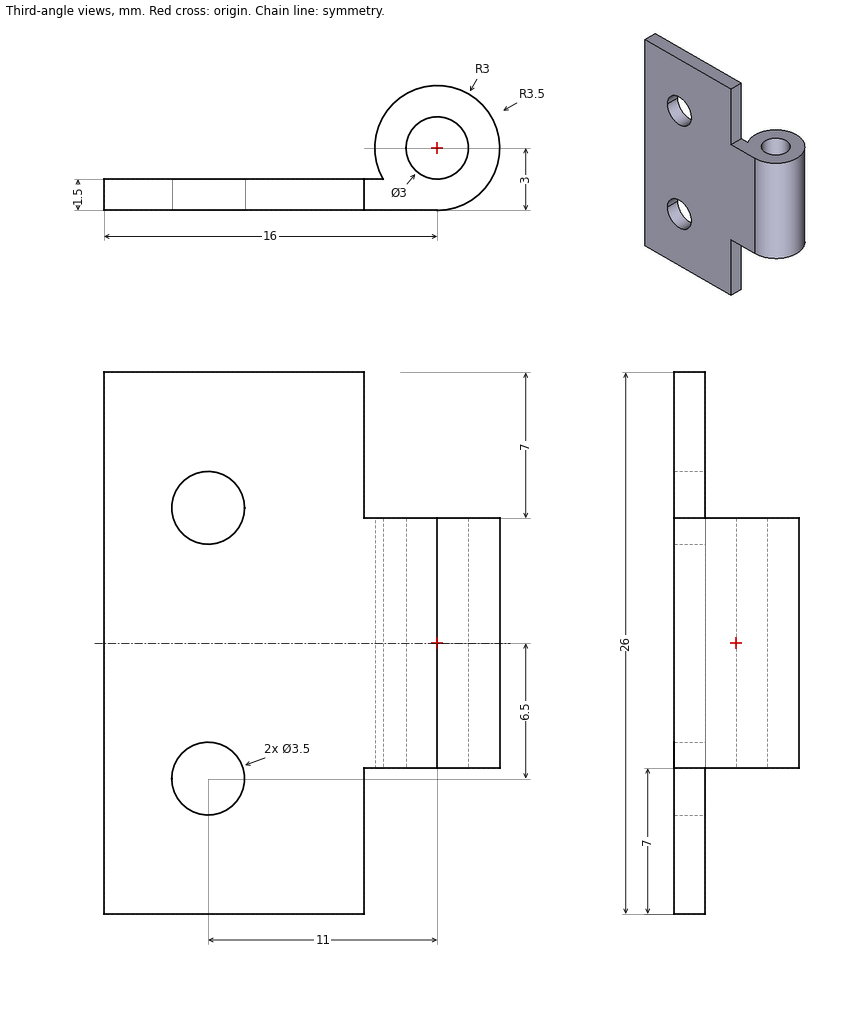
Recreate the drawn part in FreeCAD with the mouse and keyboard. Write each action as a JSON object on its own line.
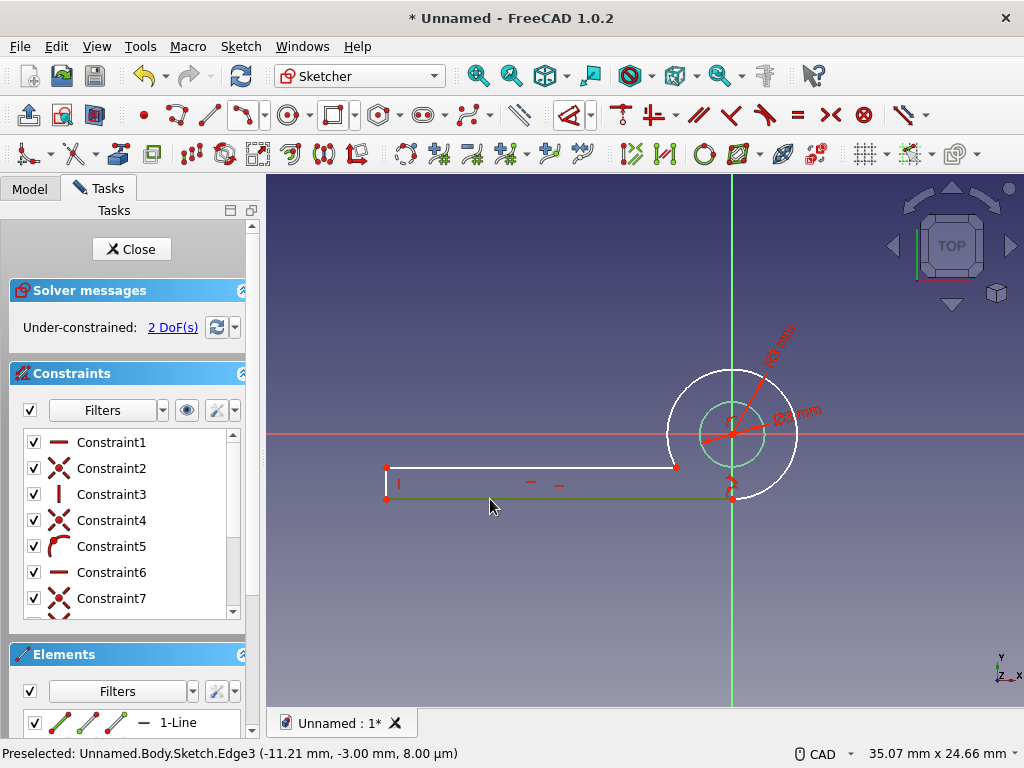
{"action": "left_click", "coordinate": [590, 116]}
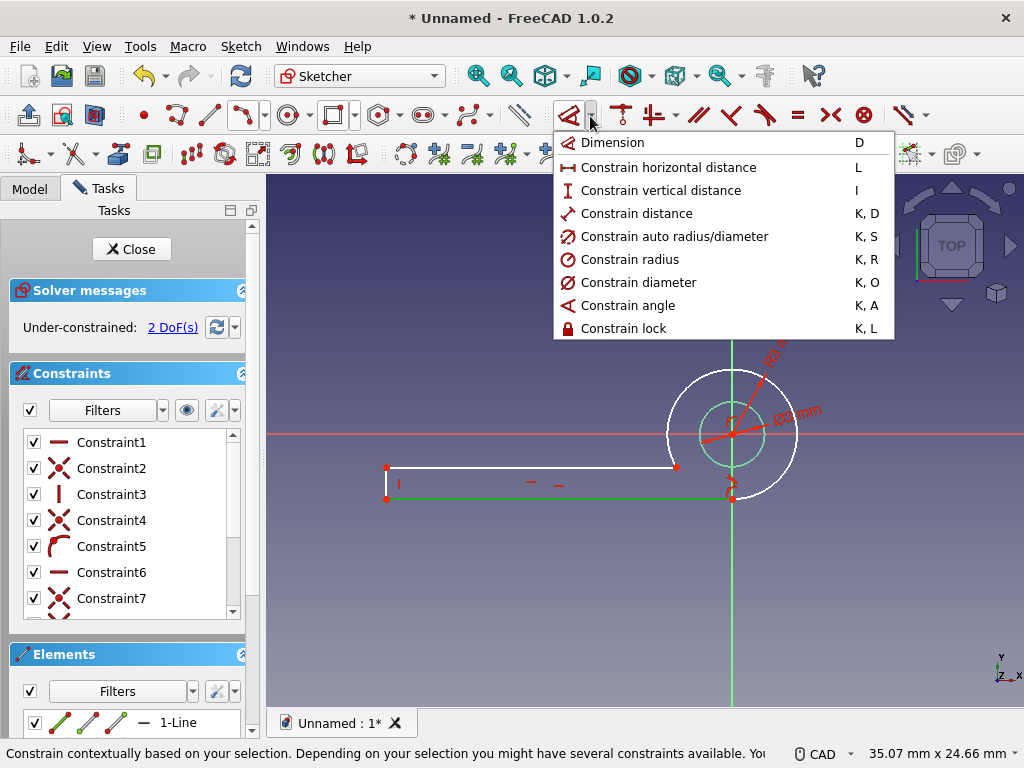
{"action": "left_click", "coordinate": [724, 168]}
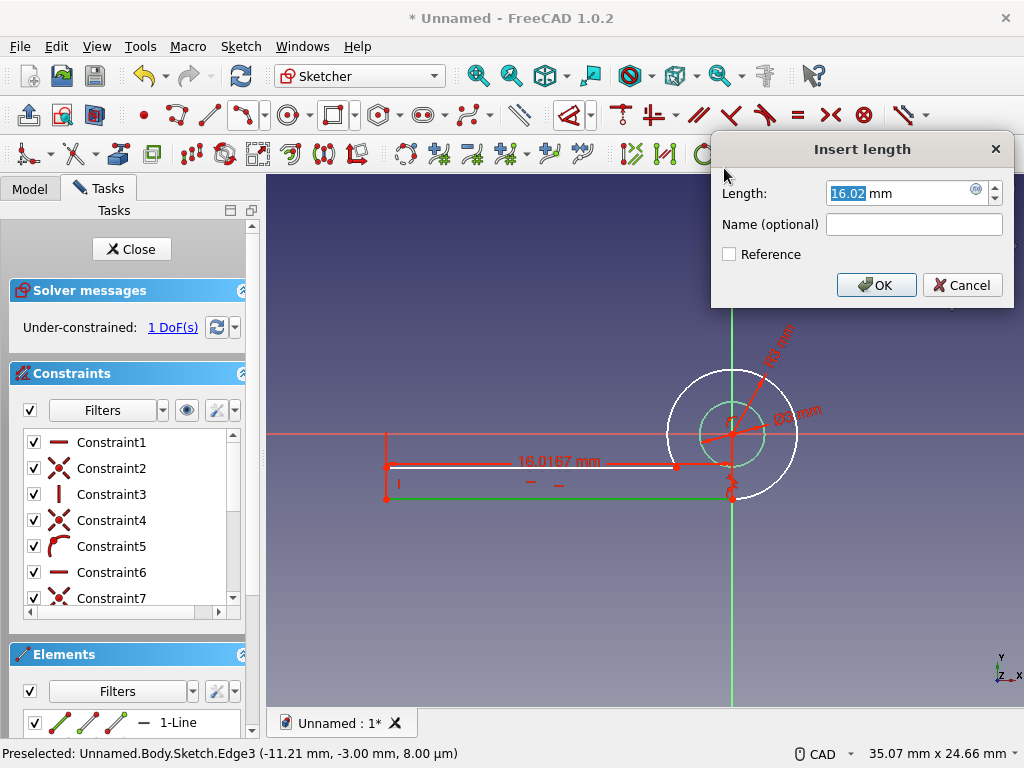
{"action": "type", "text": "16"}
{"action": "key", "text": "Return"}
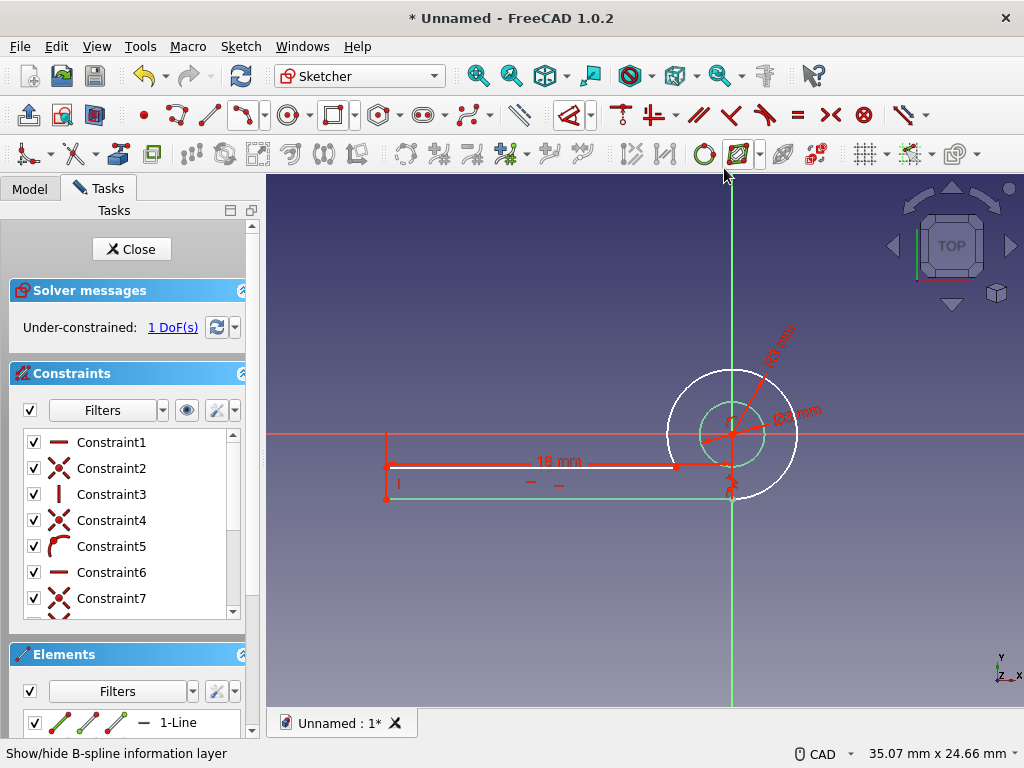
{"action": "scroll", "coordinate": [386, 477], "scroll_direction": "up", "scroll_amount": 2}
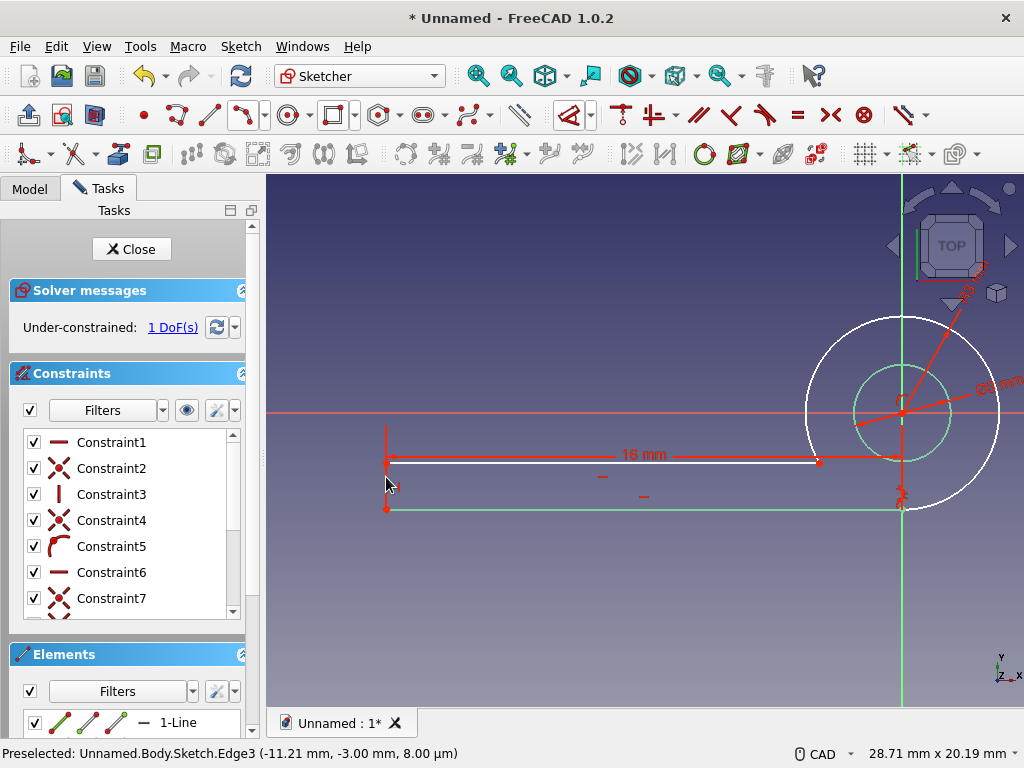
{"action": "left_click", "coordinate": [386, 477]}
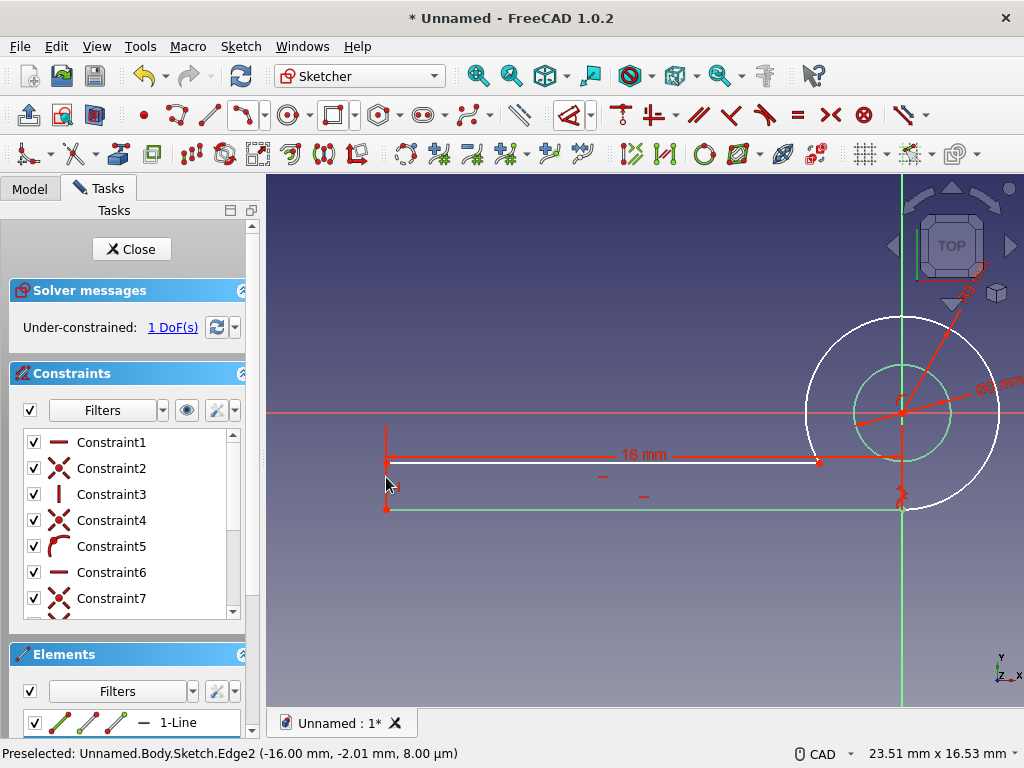
{"action": "left_click", "coordinate": [590, 116]}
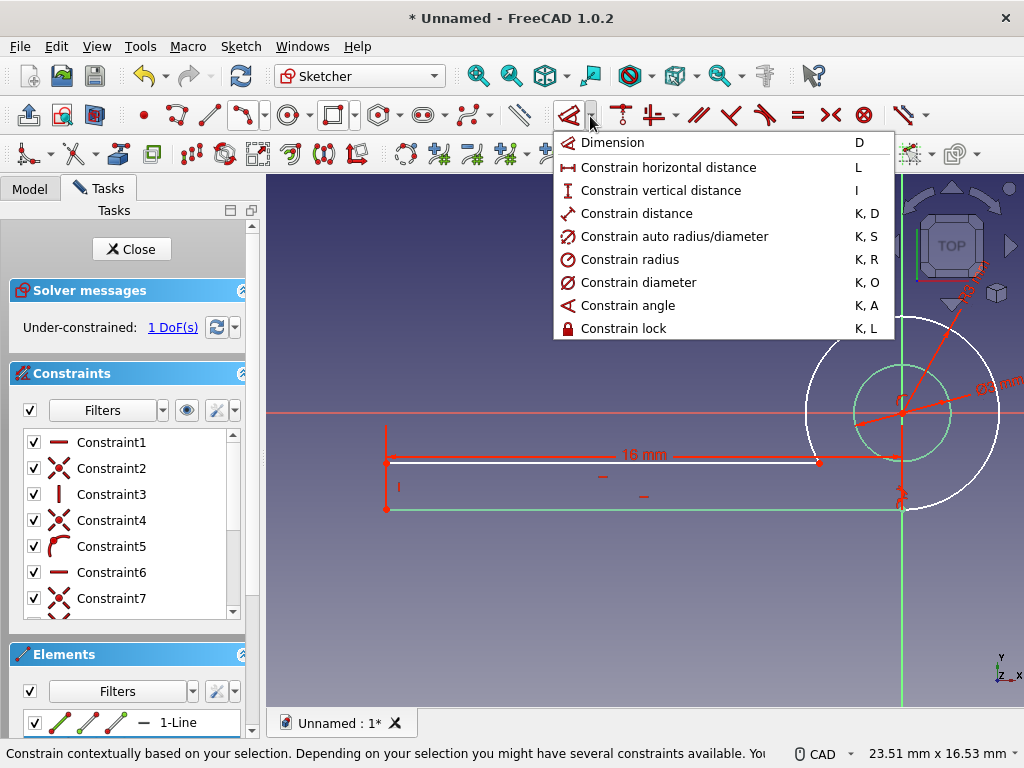
{"action": "left_click", "coordinate": [724, 190]}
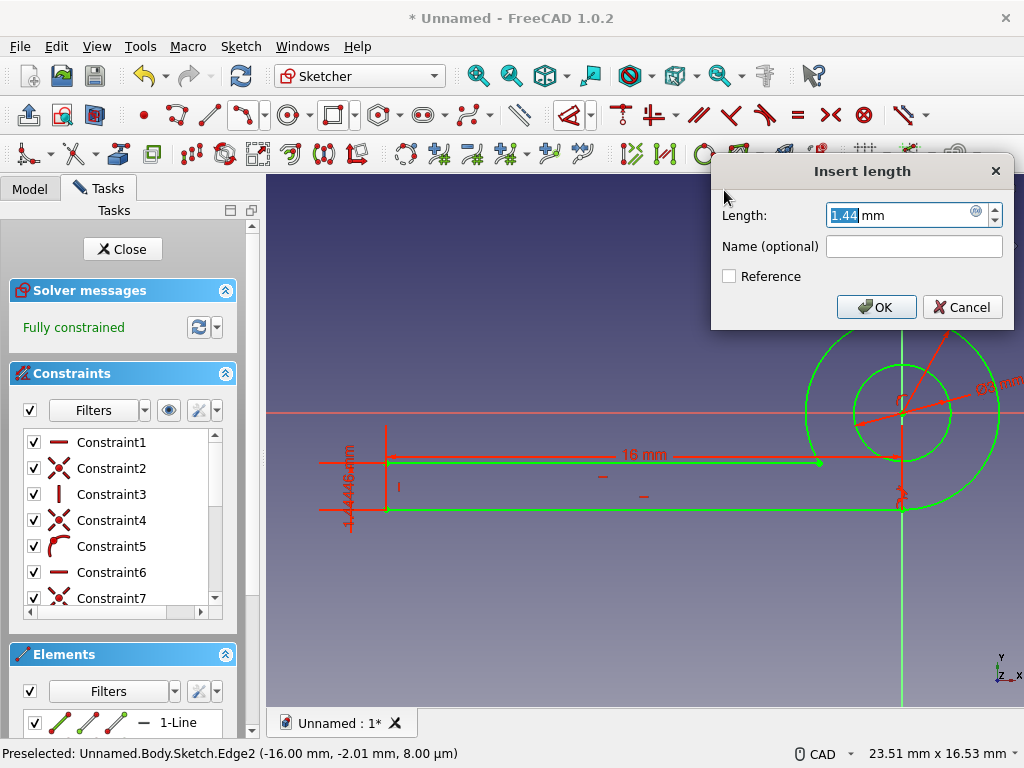
{"action": "type", "text": "1.5"}
{"action": "key", "text": "Return"}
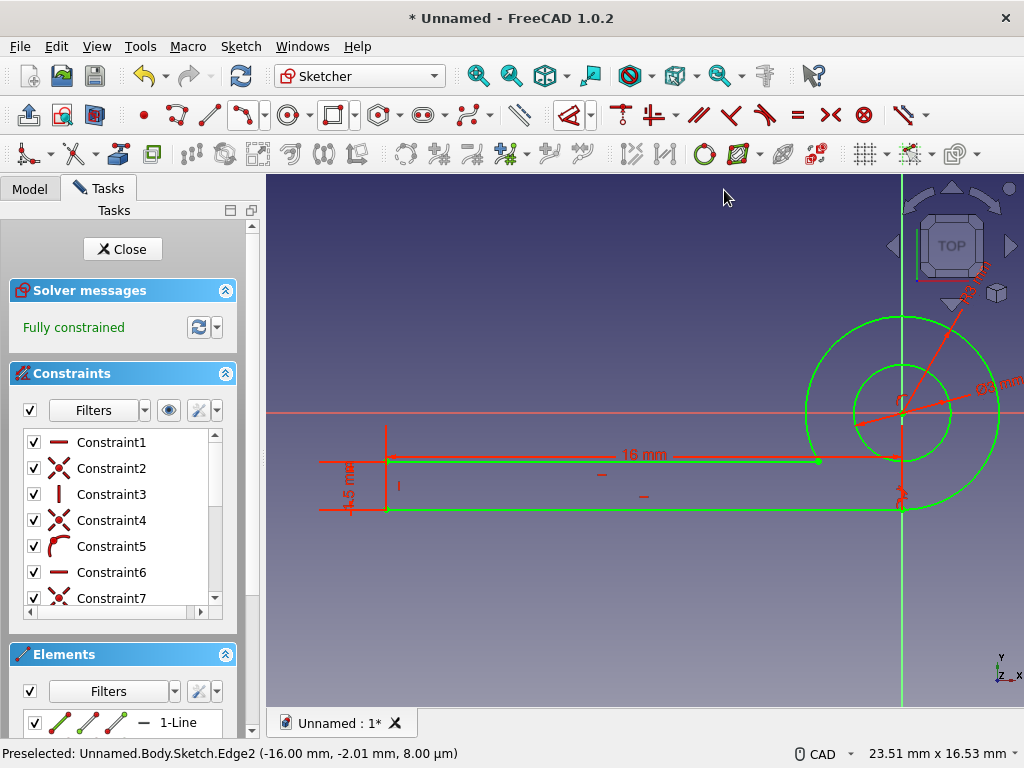
{"action": "left_click", "coordinate": [123, 249]}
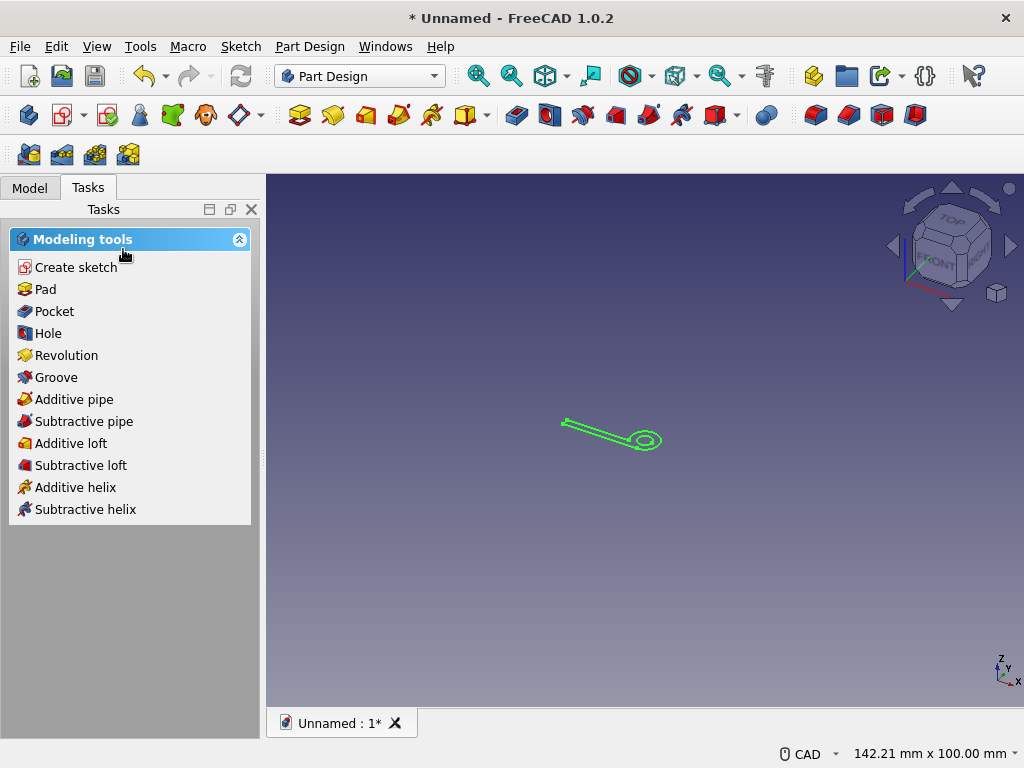
{"action": "left_click", "coordinate": [300, 116]}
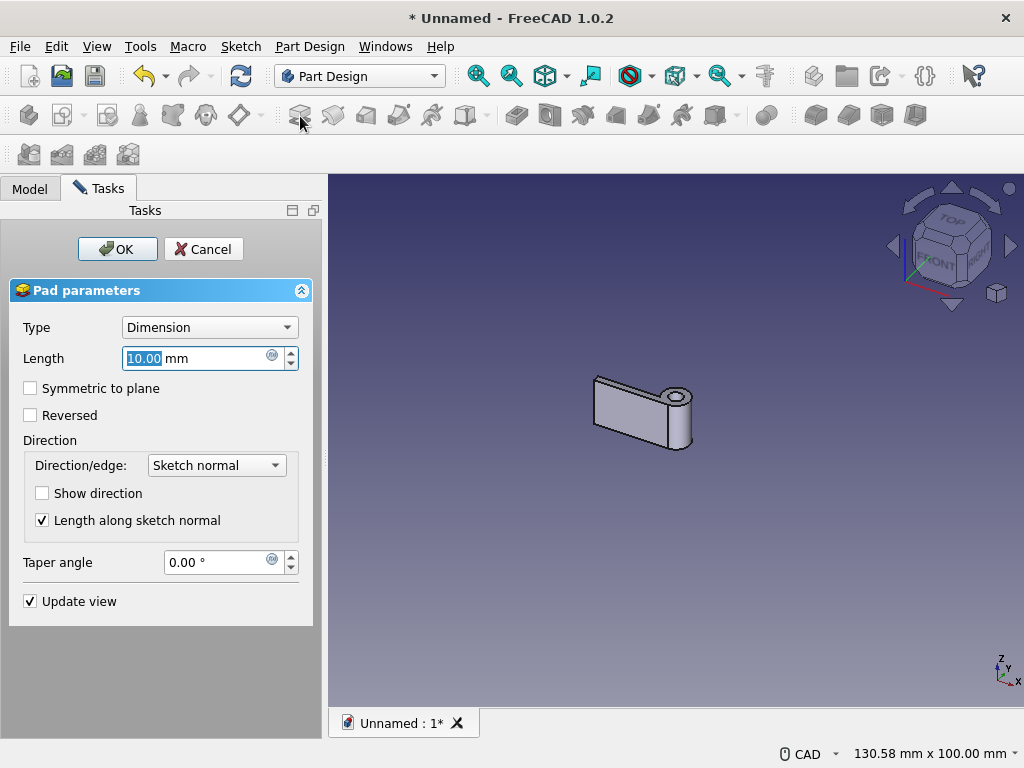
{"action": "type", "text": "26"}
{"action": "key", "text": "Tab"}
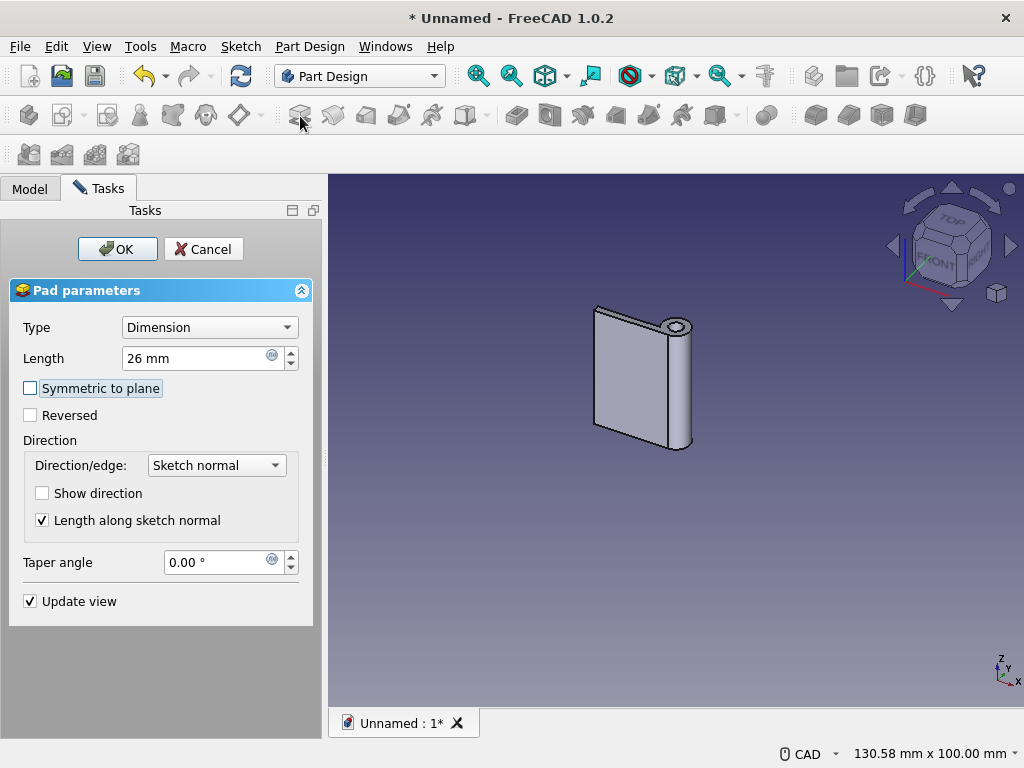
{"action": "left_click", "coordinate": [31, 388]}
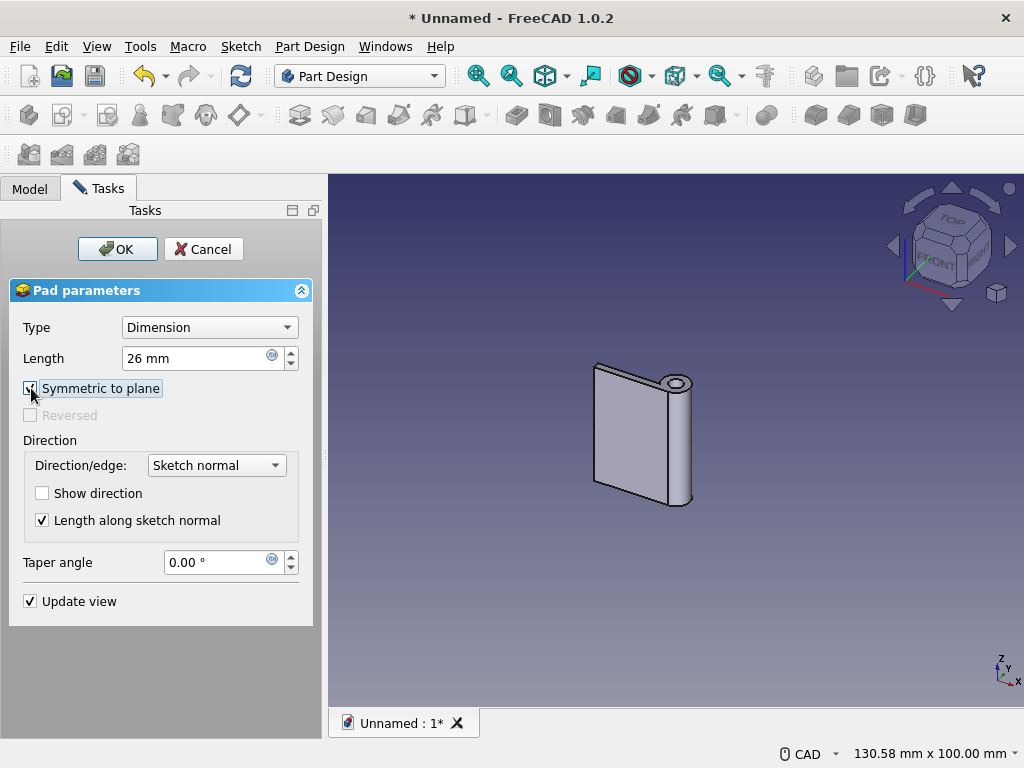
{"action": "left_click", "coordinate": [118, 249]}